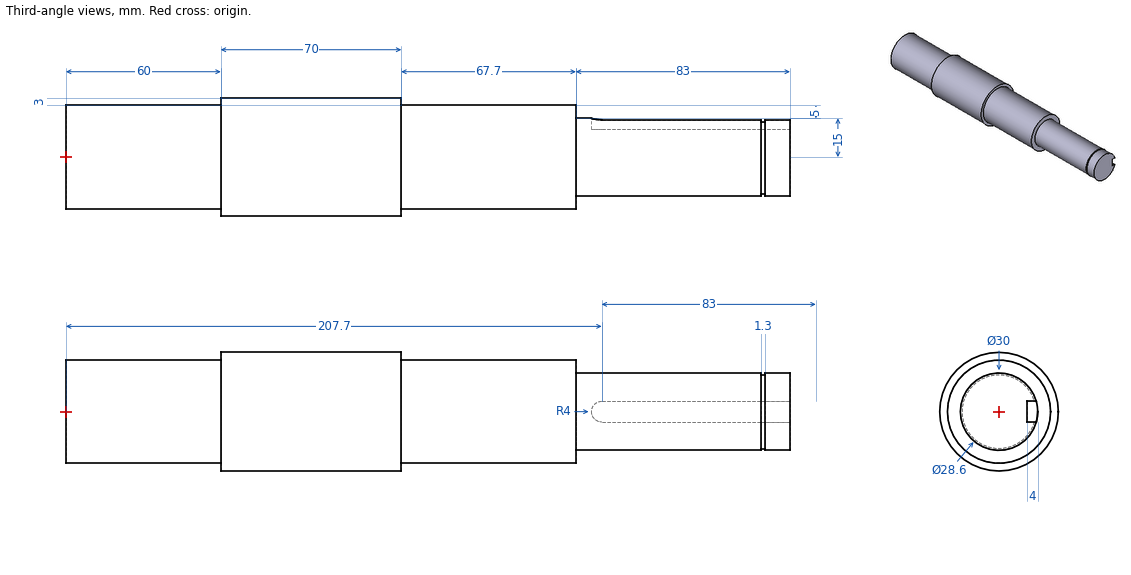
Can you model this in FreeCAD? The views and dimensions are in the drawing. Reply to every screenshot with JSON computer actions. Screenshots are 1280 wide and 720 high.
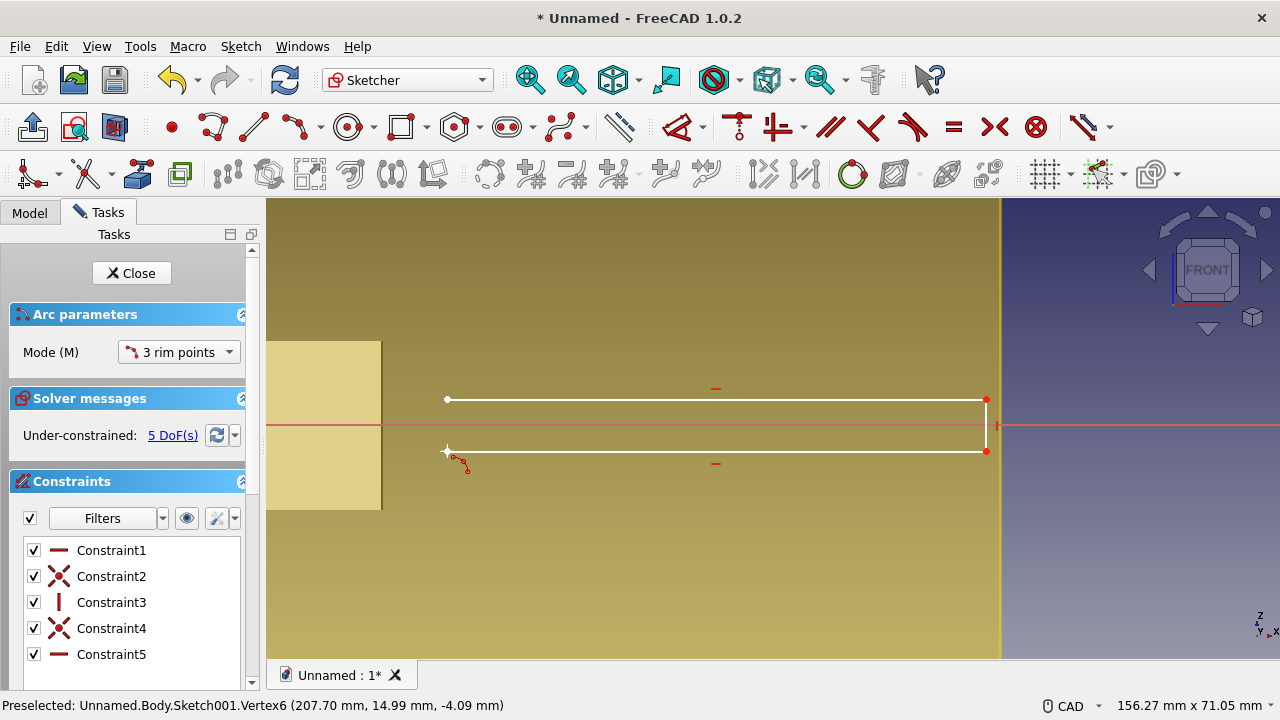
{"action": "left_click", "coordinate": [447, 452]}
{"action": "left_click", "coordinate": [447, 400]}
{"action": "left_click", "coordinate": [426, 410]}
{"action": "key", "text": "Escape"}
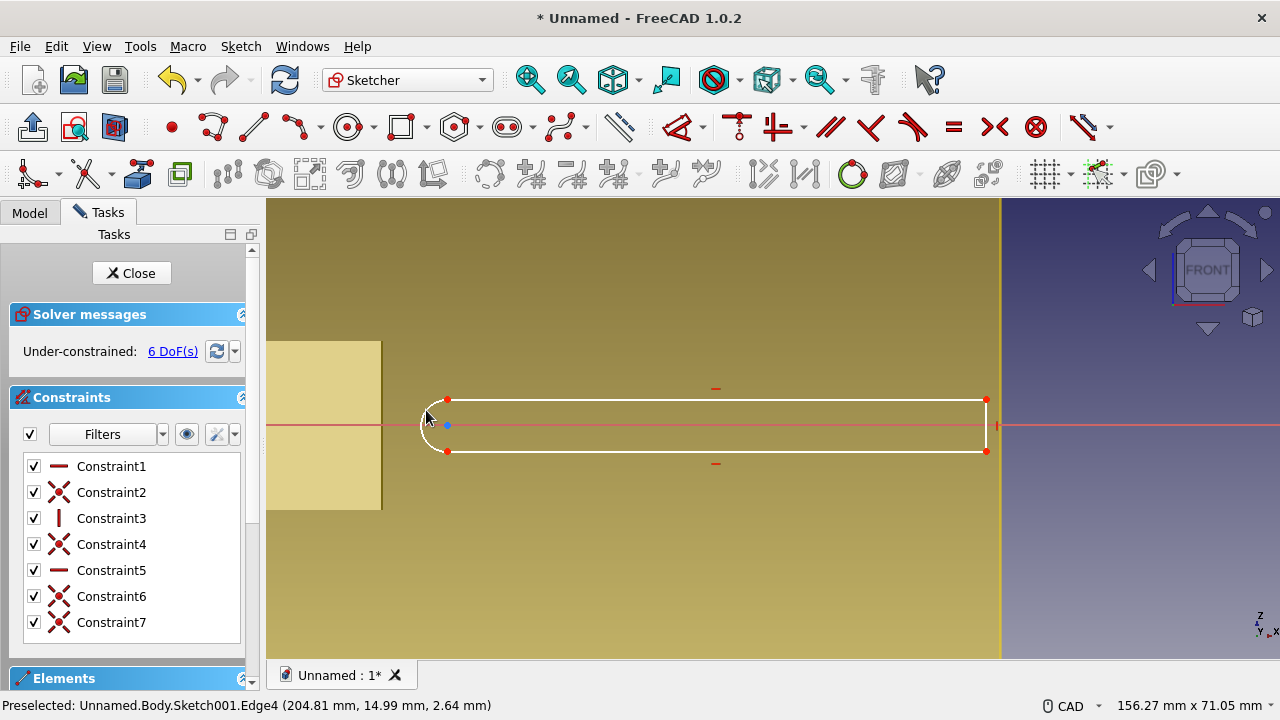
{"action": "left_click", "coordinate": [609, 400]}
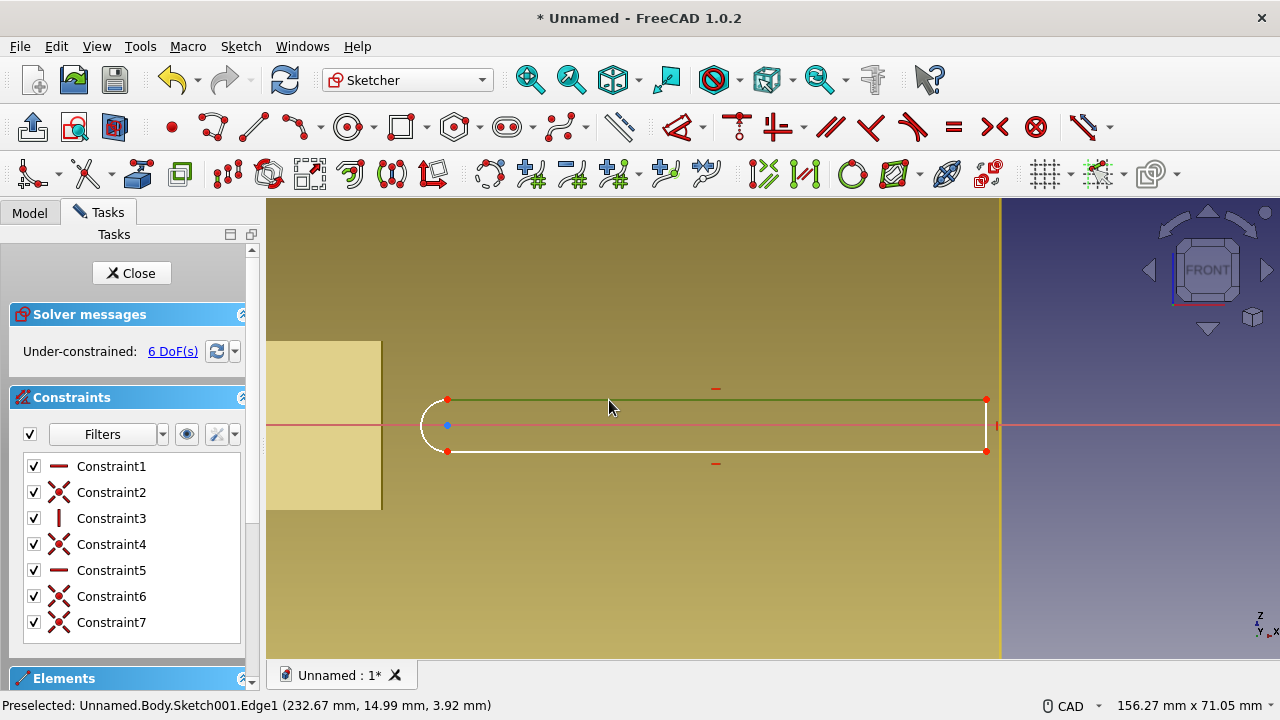
{"action": "left_click", "coordinate": [426, 411]}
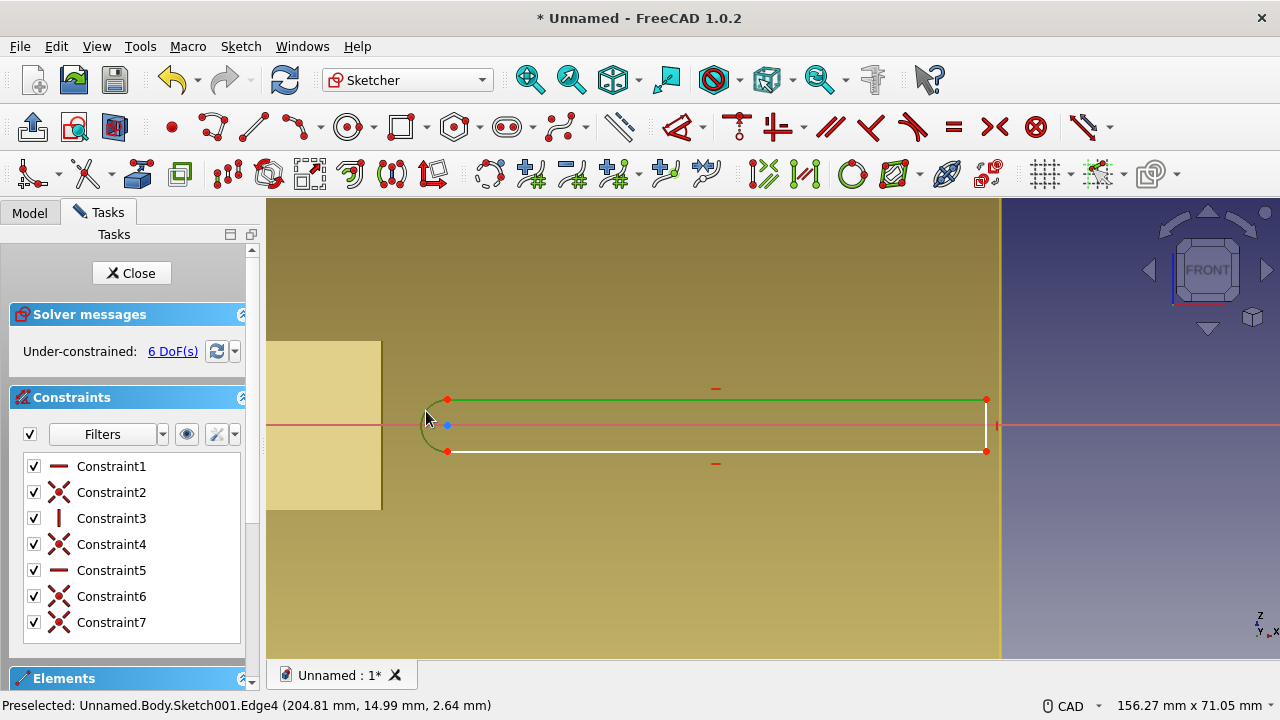
{"action": "left_click", "coordinate": [913, 128]}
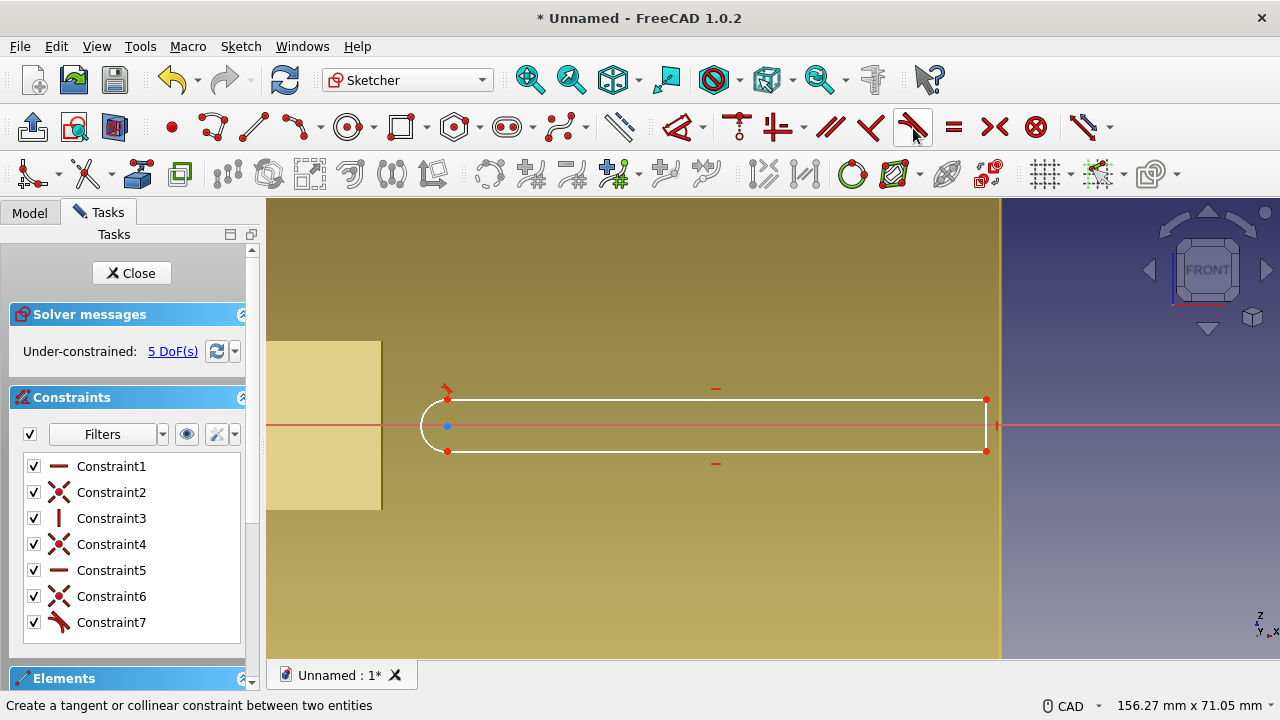
{"action": "left_click", "coordinate": [824, 452]}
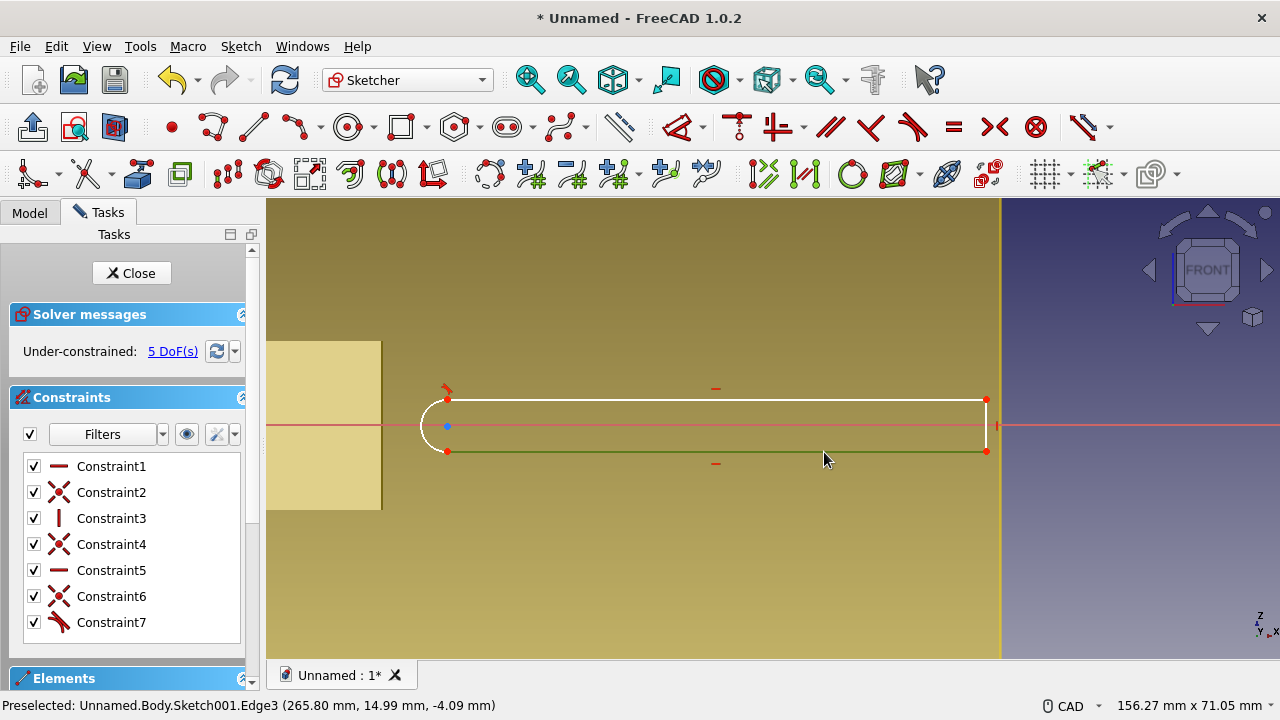
{"action": "left_click", "coordinate": [426, 411]}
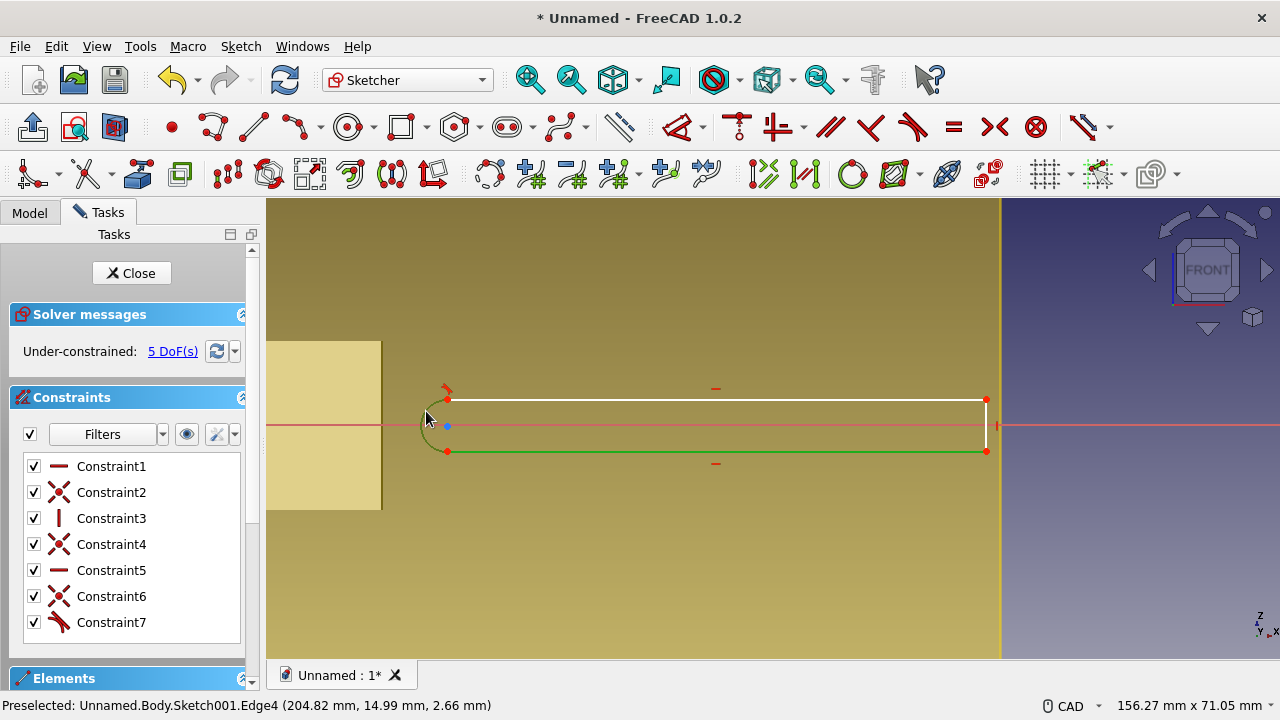
{"action": "key", "text": "t"}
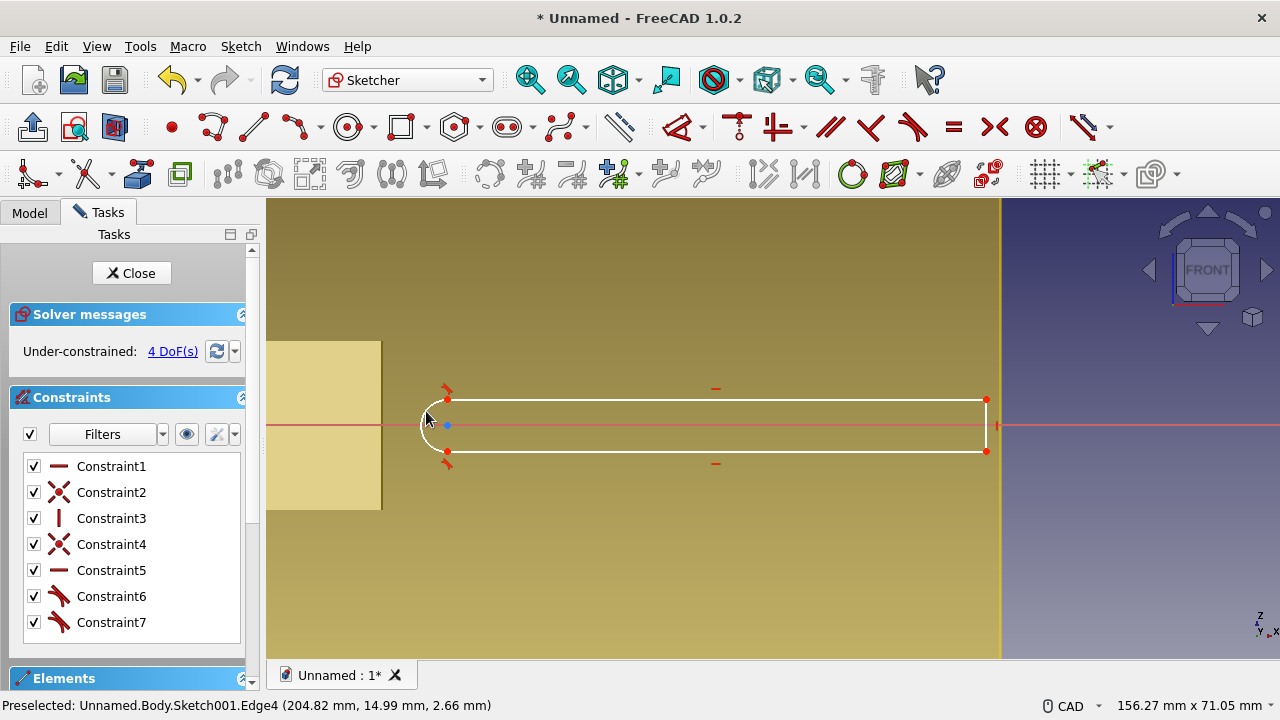
{"action": "left_click", "coordinate": [447, 426]}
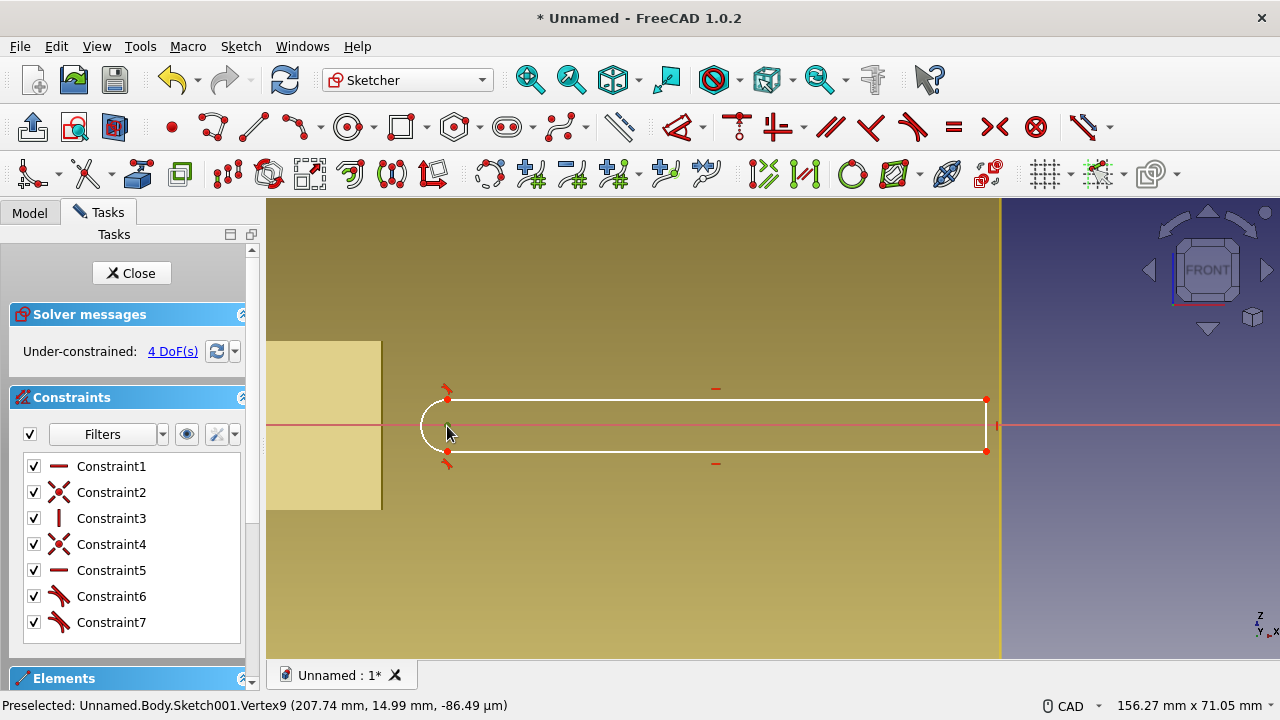
{"action": "left_click", "coordinate": [353, 425]}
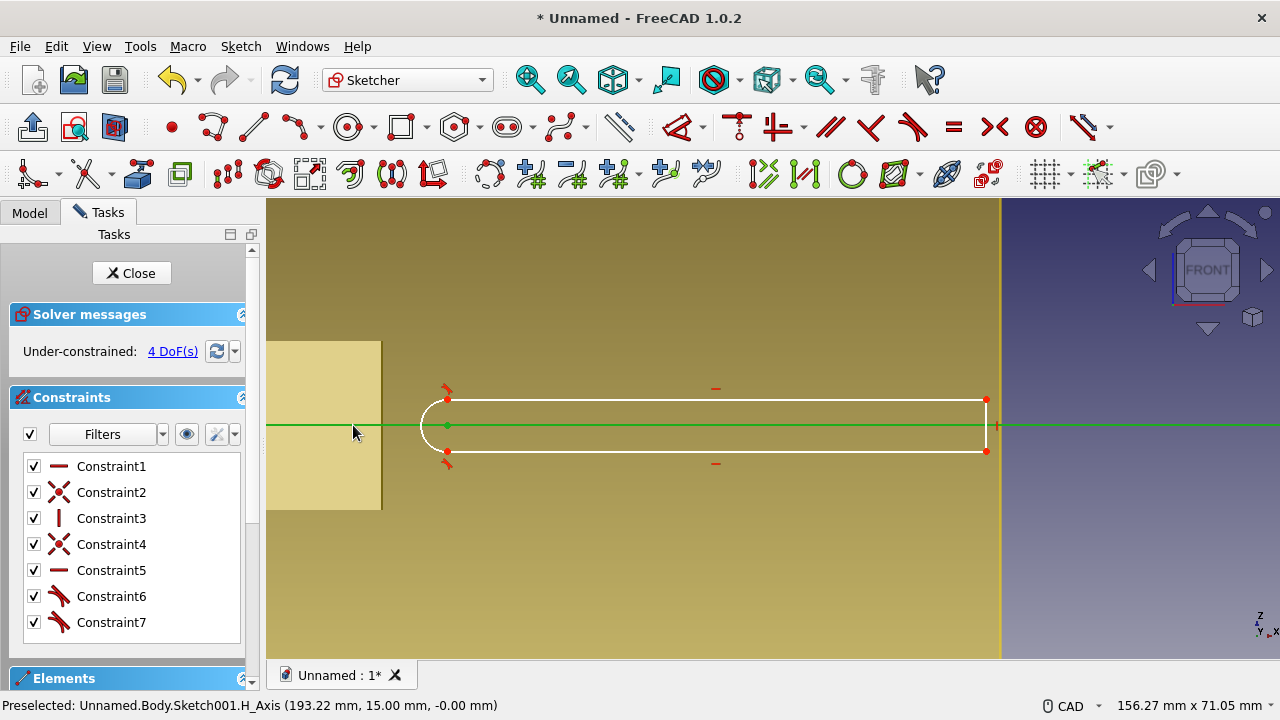
{"action": "key", "text": "c"}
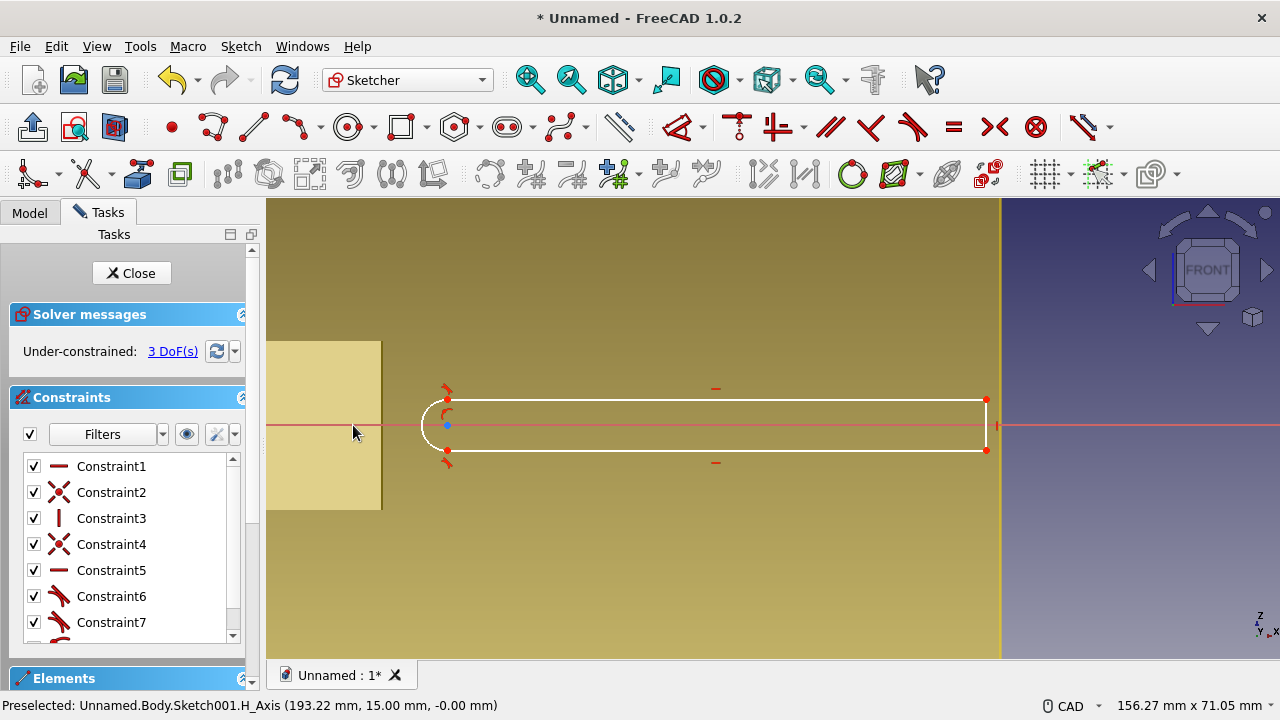
{"action": "left_click", "coordinate": [676, 128]}